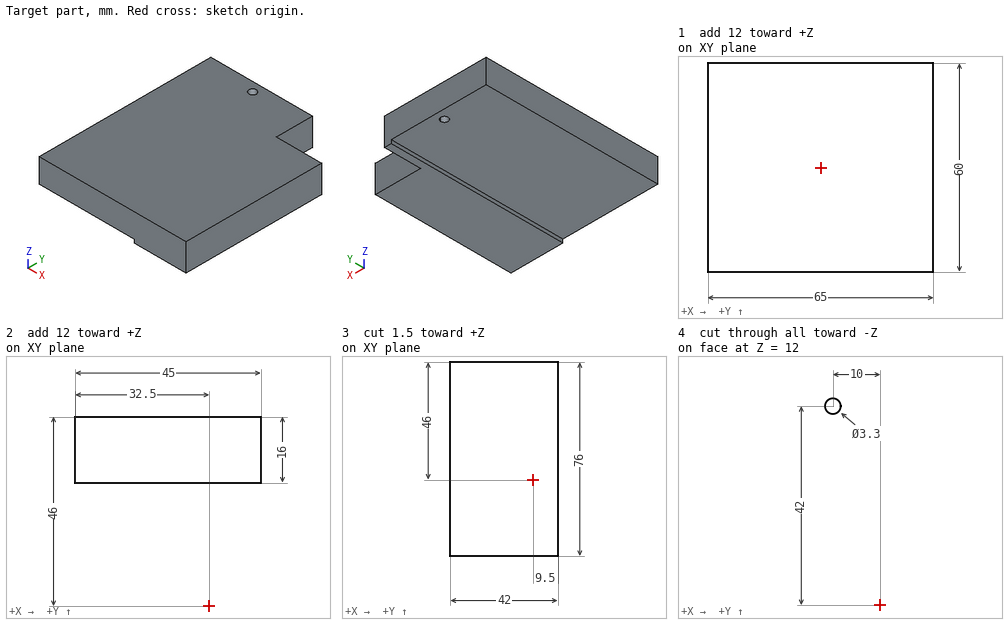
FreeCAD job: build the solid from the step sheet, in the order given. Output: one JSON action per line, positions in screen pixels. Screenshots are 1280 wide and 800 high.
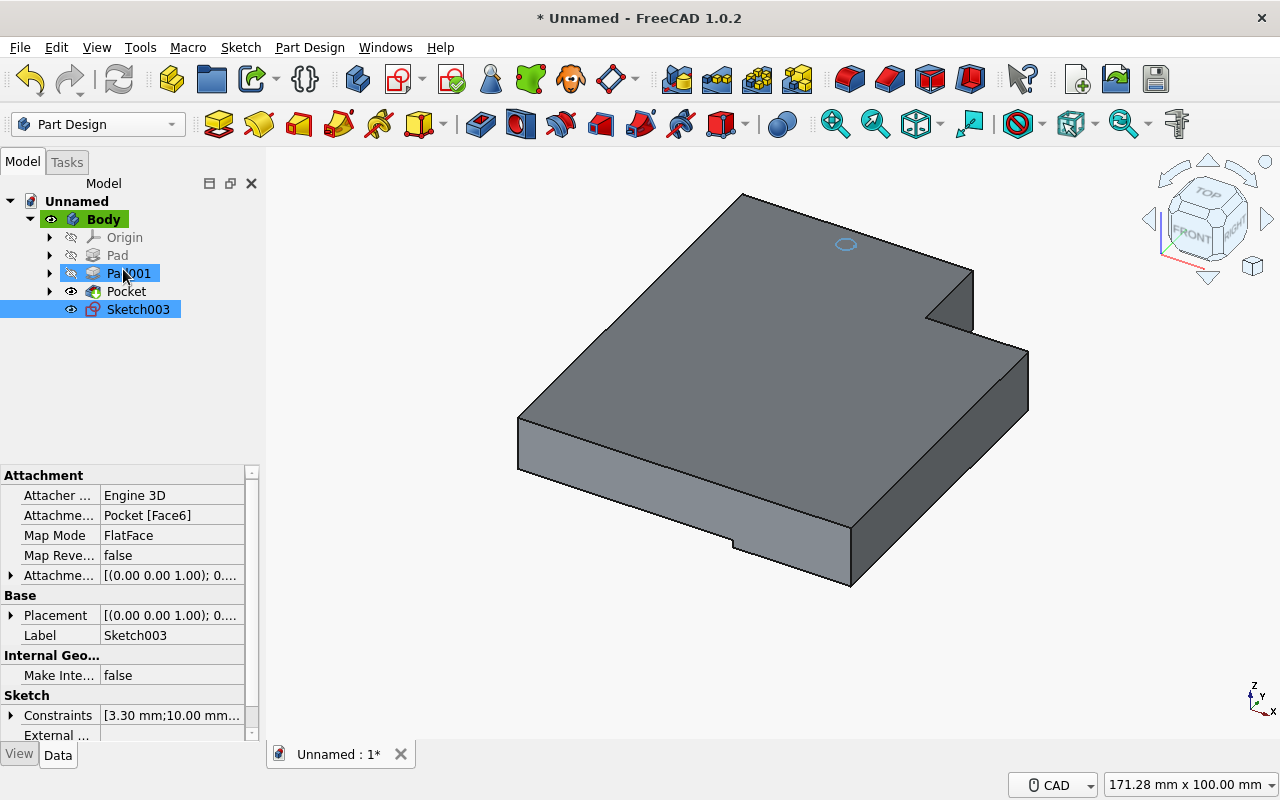
{"action": "left_click", "coordinate": [482, 124]}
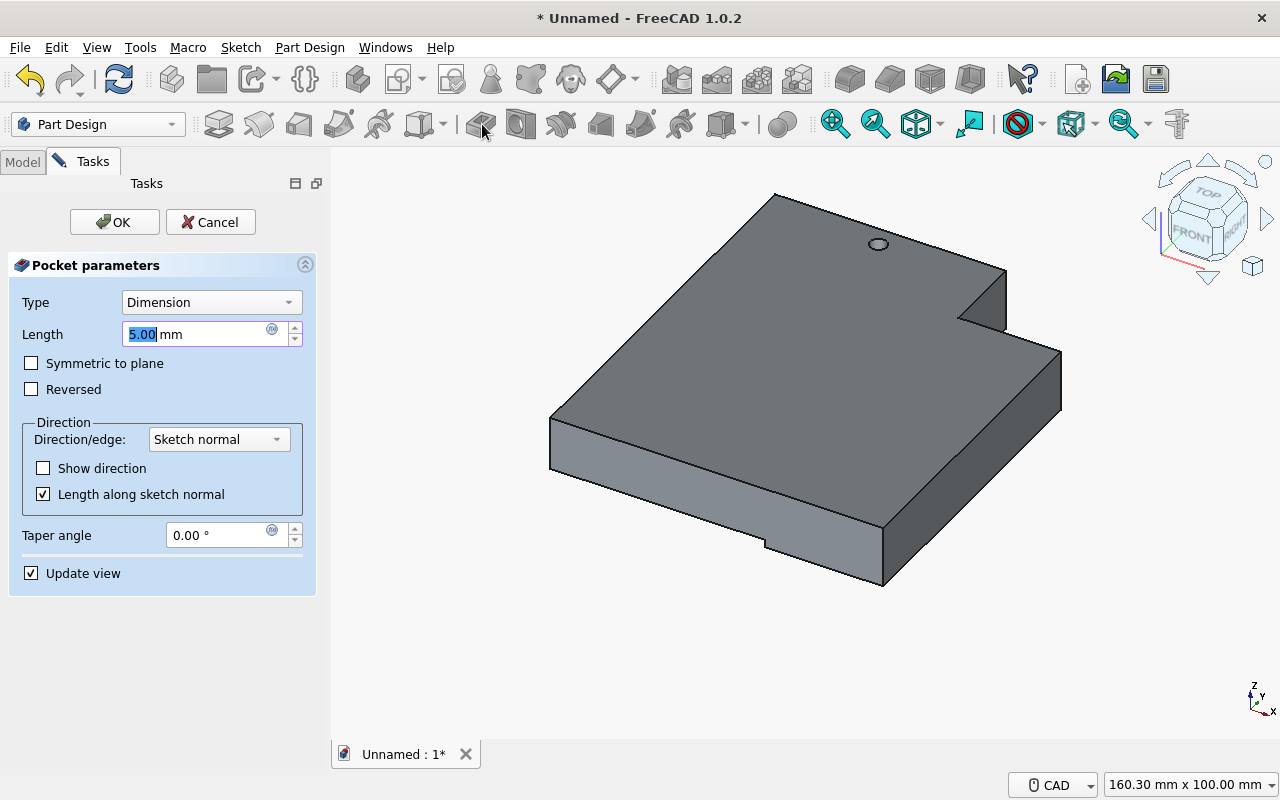
{"action": "left_click", "coordinate": [212, 302]}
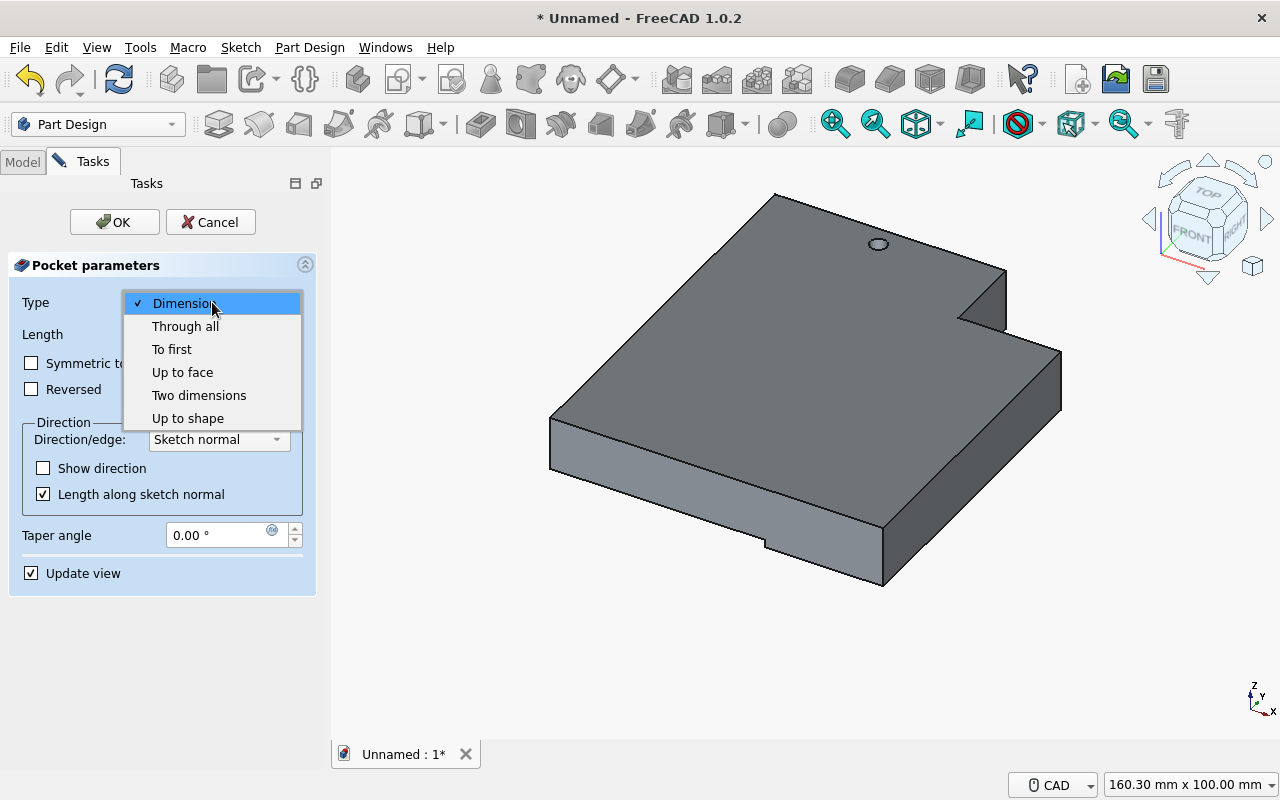
{"action": "left_click", "coordinate": [212, 326]}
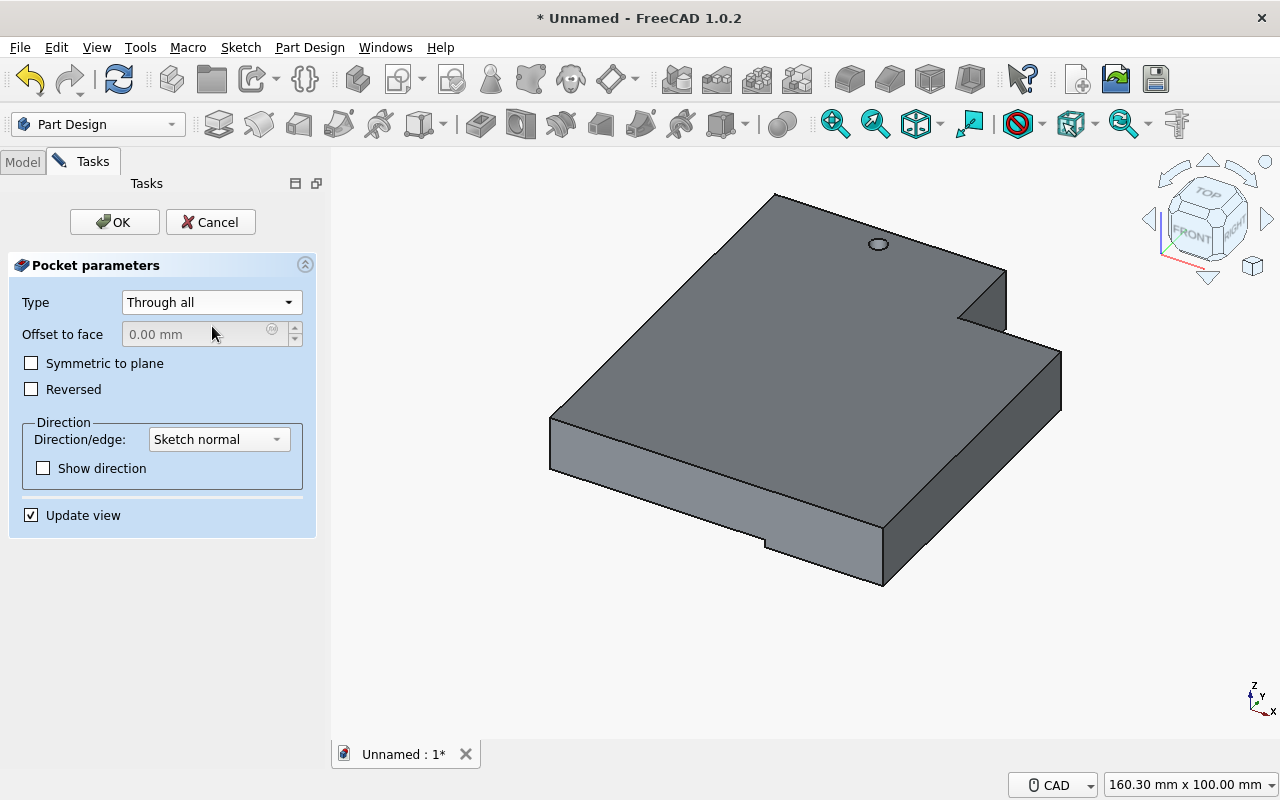
{"action": "left_click", "coordinate": [115, 222]}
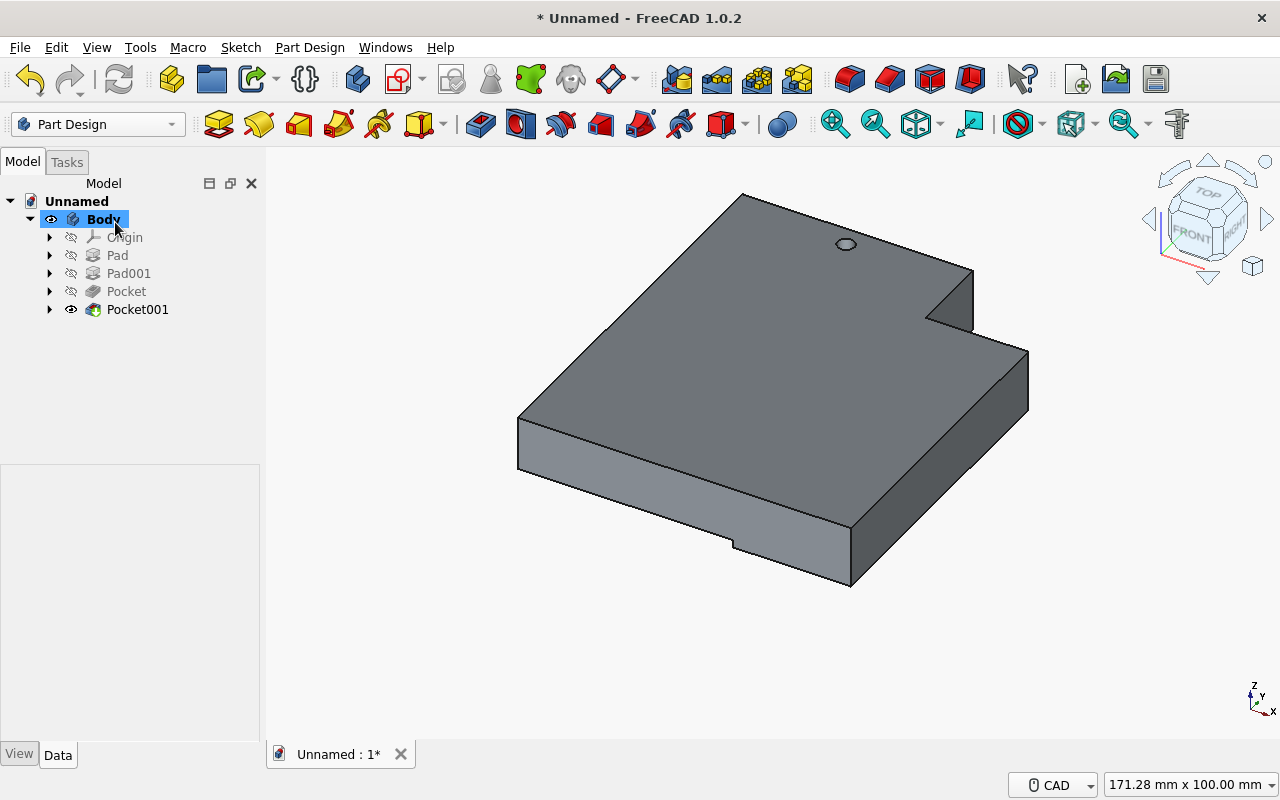
{"action": "key", "text": "0"}